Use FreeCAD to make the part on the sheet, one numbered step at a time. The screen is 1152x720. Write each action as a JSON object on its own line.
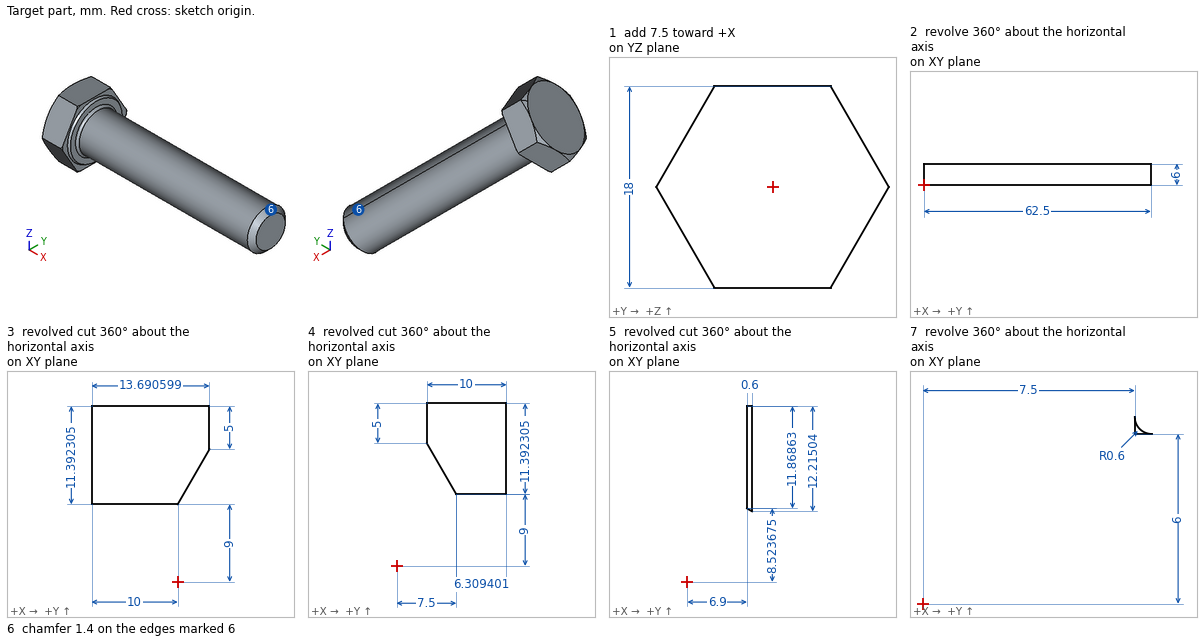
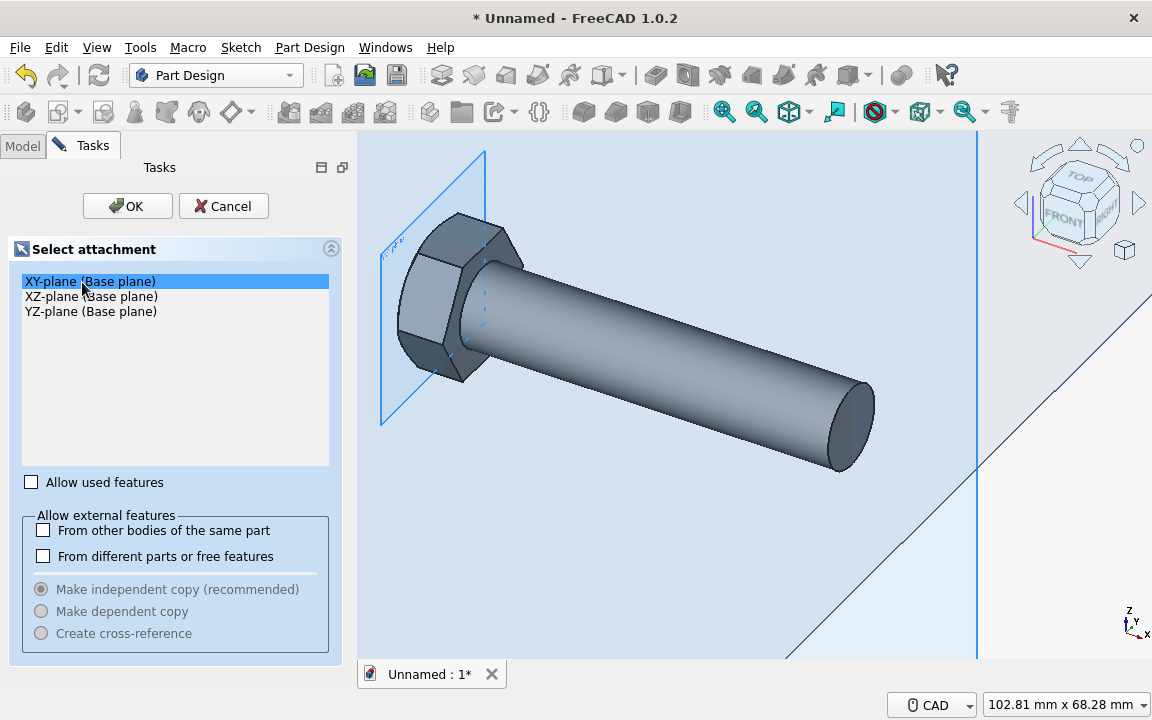
{"action": "left_click", "coordinate": [128, 206]}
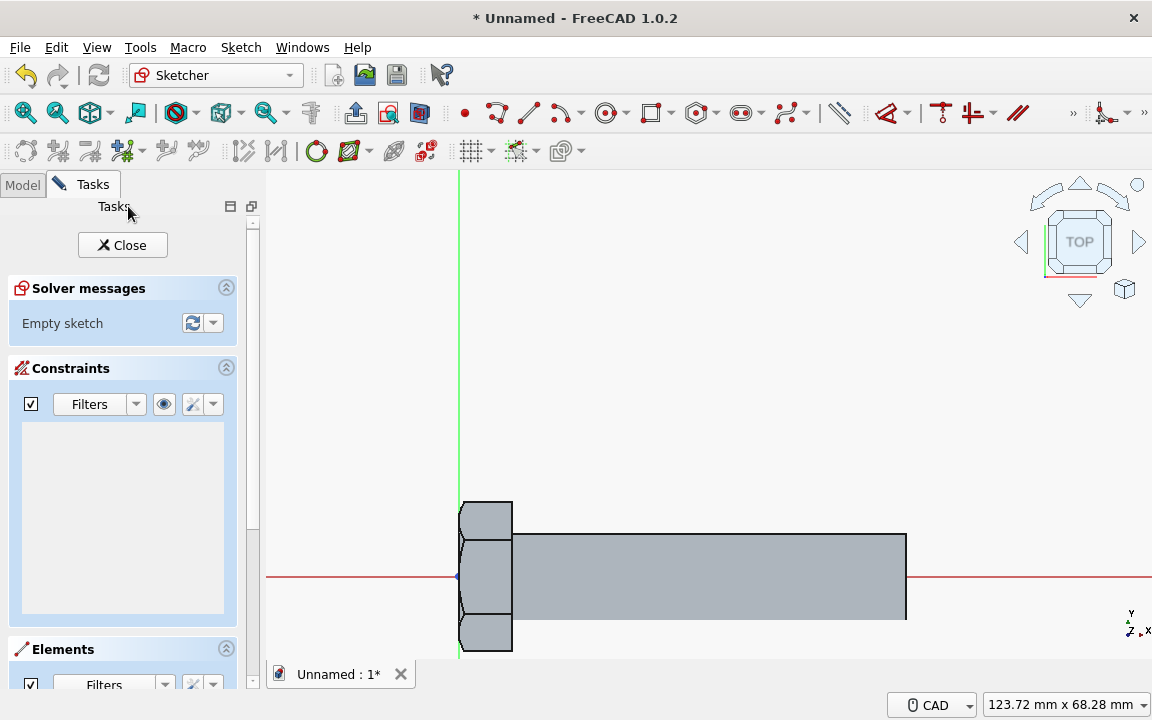
{"action": "key", "text": "q s"}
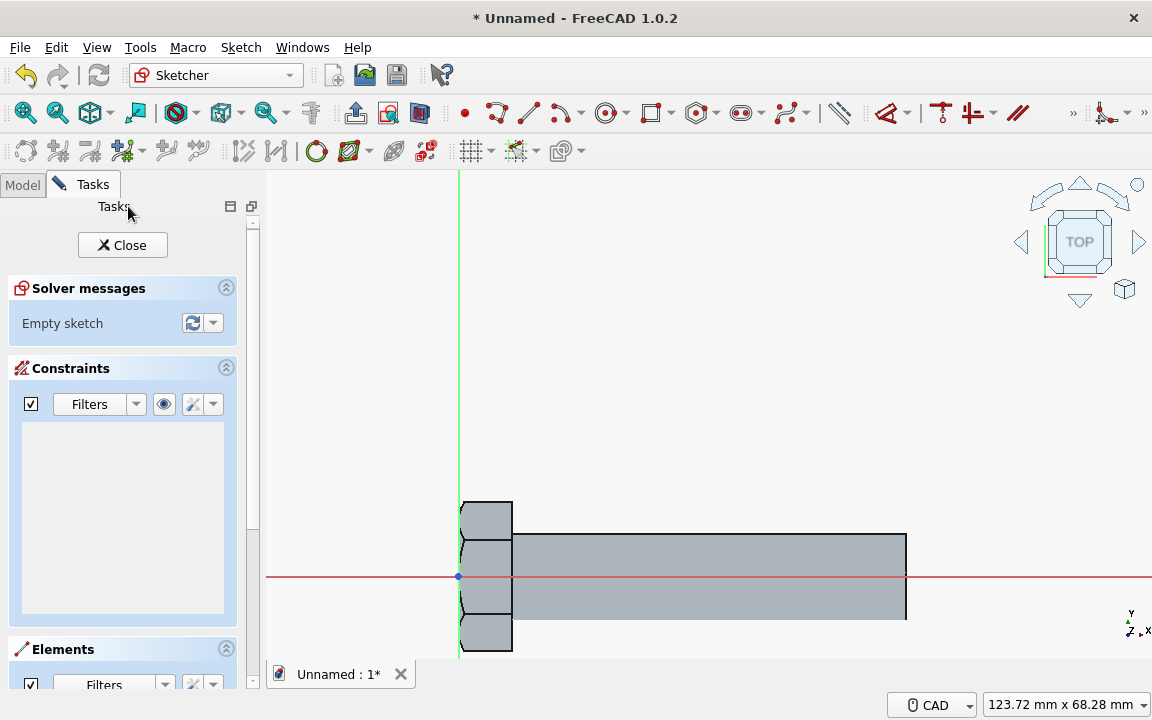
{"action": "scroll", "coordinate": [400, 577], "scroll_direction": "up", "scroll_amount": 4}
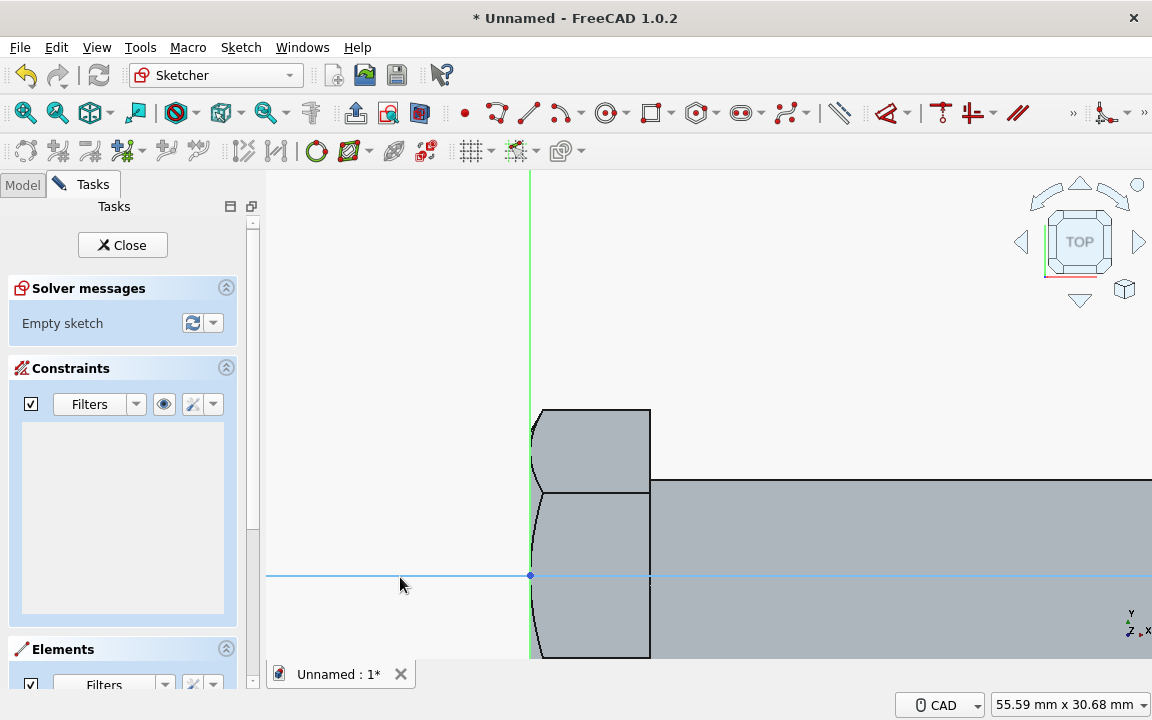
{"action": "key", "text": "g m"}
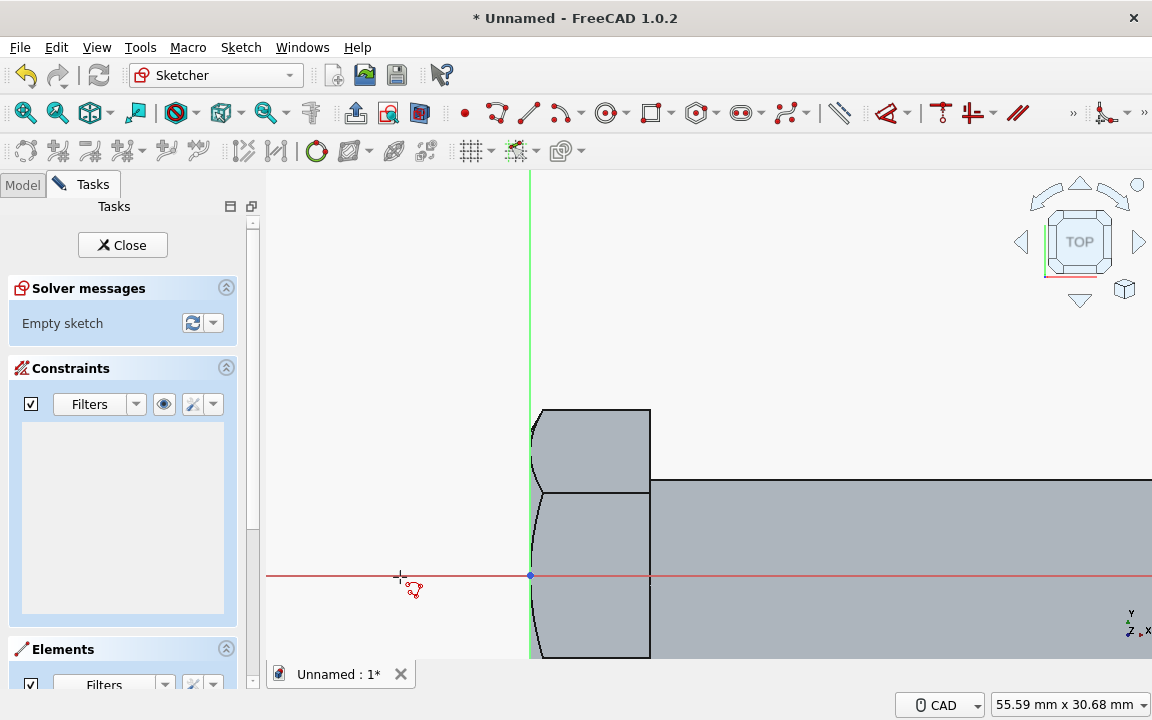
{"action": "left_click", "coordinate": [650, 432]}
{"action": "left_click", "coordinate": [750, 432]}
{"action": "left_click", "coordinate": [750, 251]}
{"action": "left_click", "coordinate": [591, 251]}
{"action": "left_click", "coordinate": [591, 330]}
{"action": "left_click", "coordinate": [650, 433]}
{"action": "key", "text": "Escape"}
{"action": "key", "text": "Escape"}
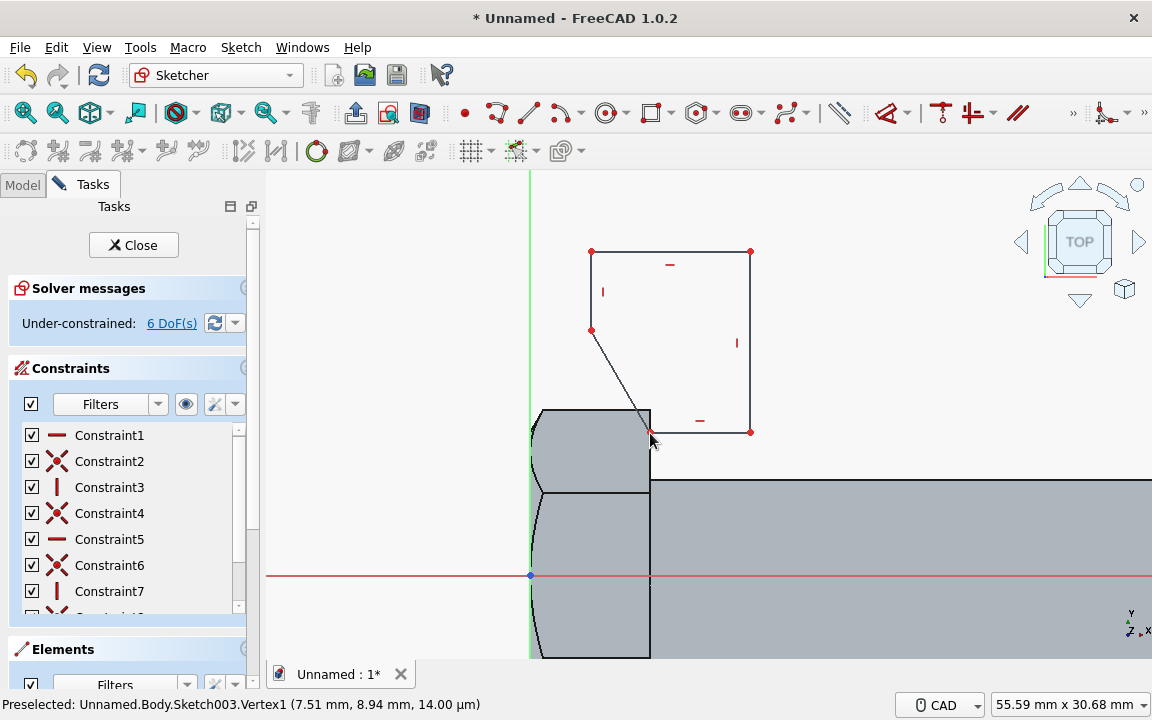
{"action": "key", "text": "d"}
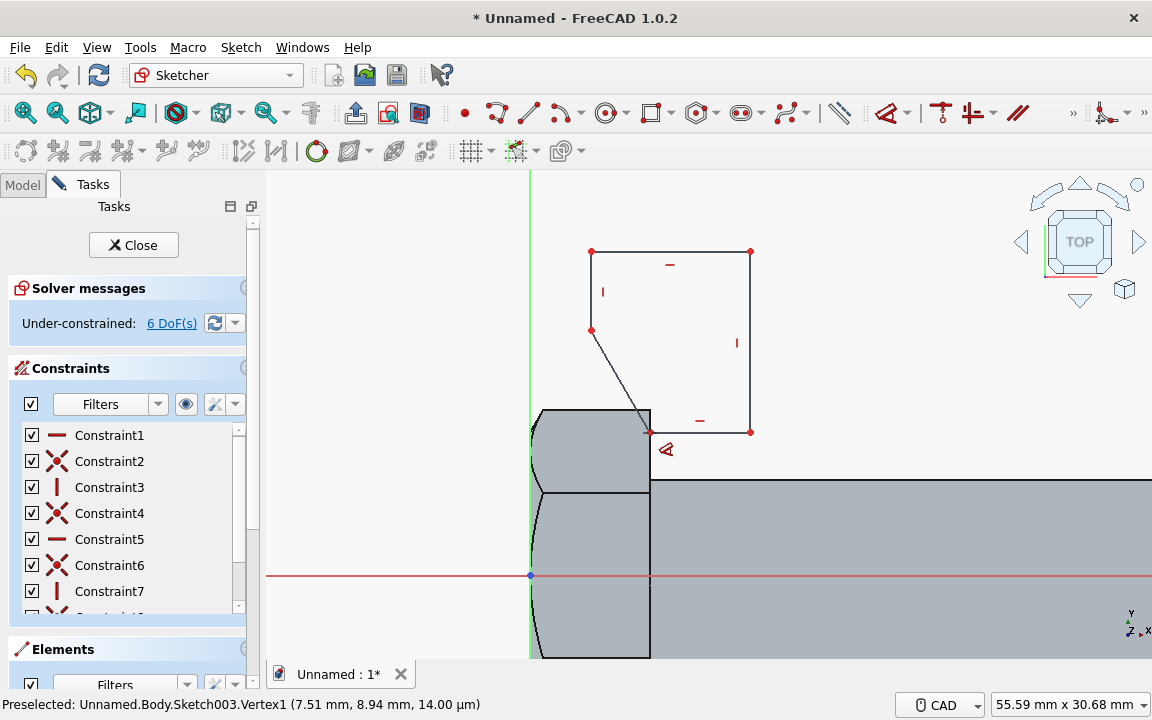
{"action": "left_click", "coordinate": [591, 276]}
{"action": "left_click", "coordinate": [557, 291]}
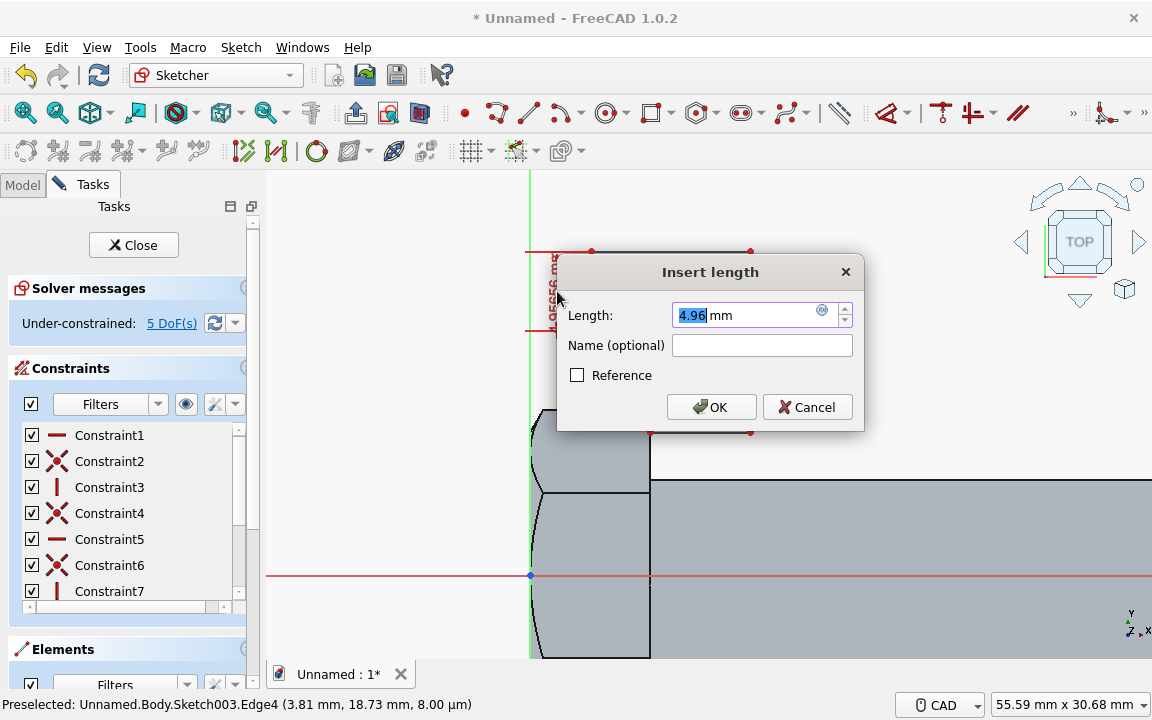
{"action": "type", "text": "5"}
{"action": "key", "text": "Return"}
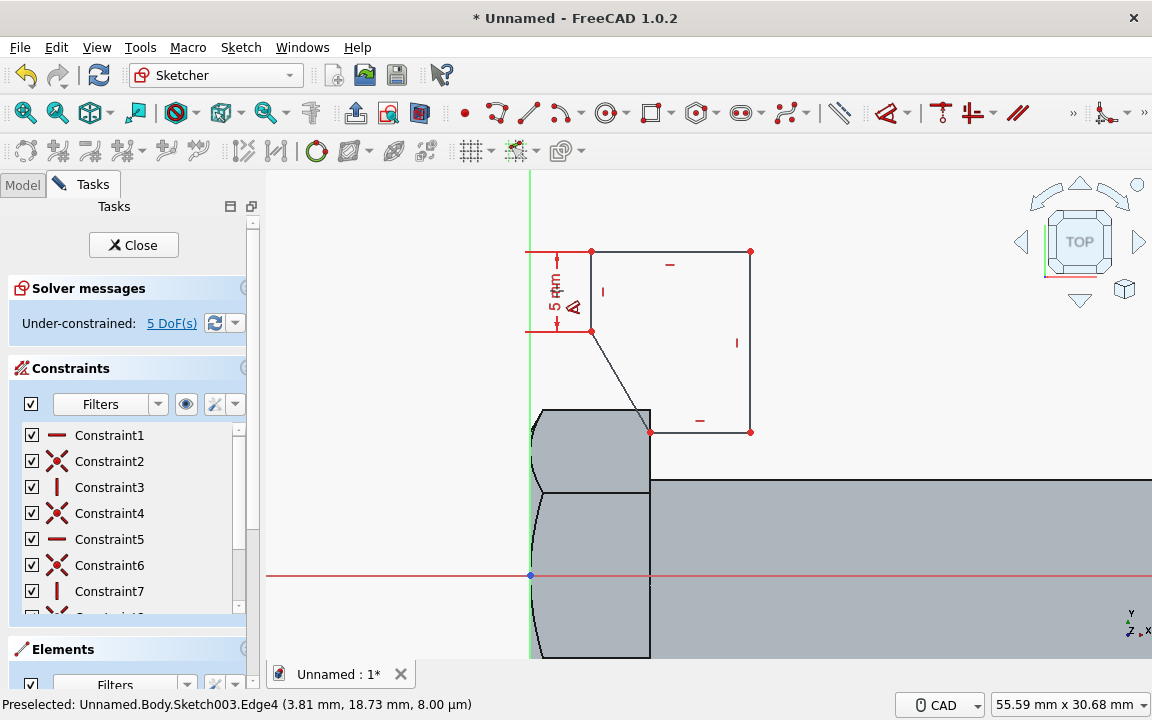
{"action": "left_click", "coordinate": [702, 252]}
{"action": "left_click", "coordinate": [670, 218]}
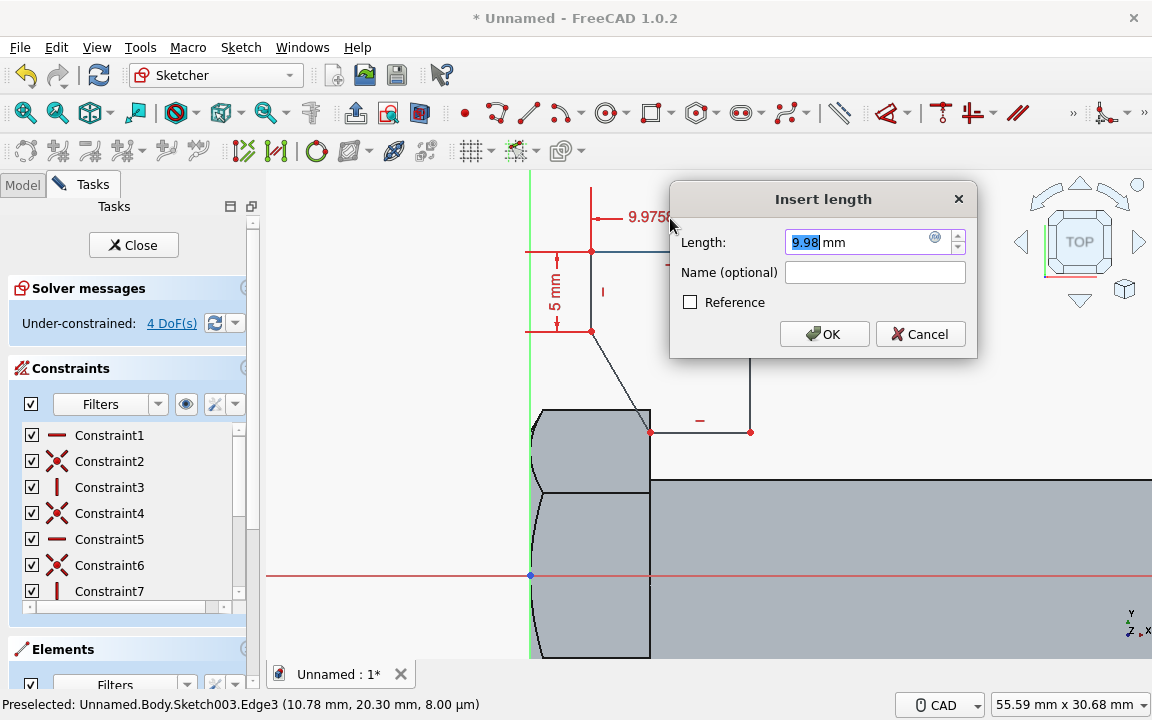
{"action": "type", "text": "10"}
{"action": "key", "text": "Return"}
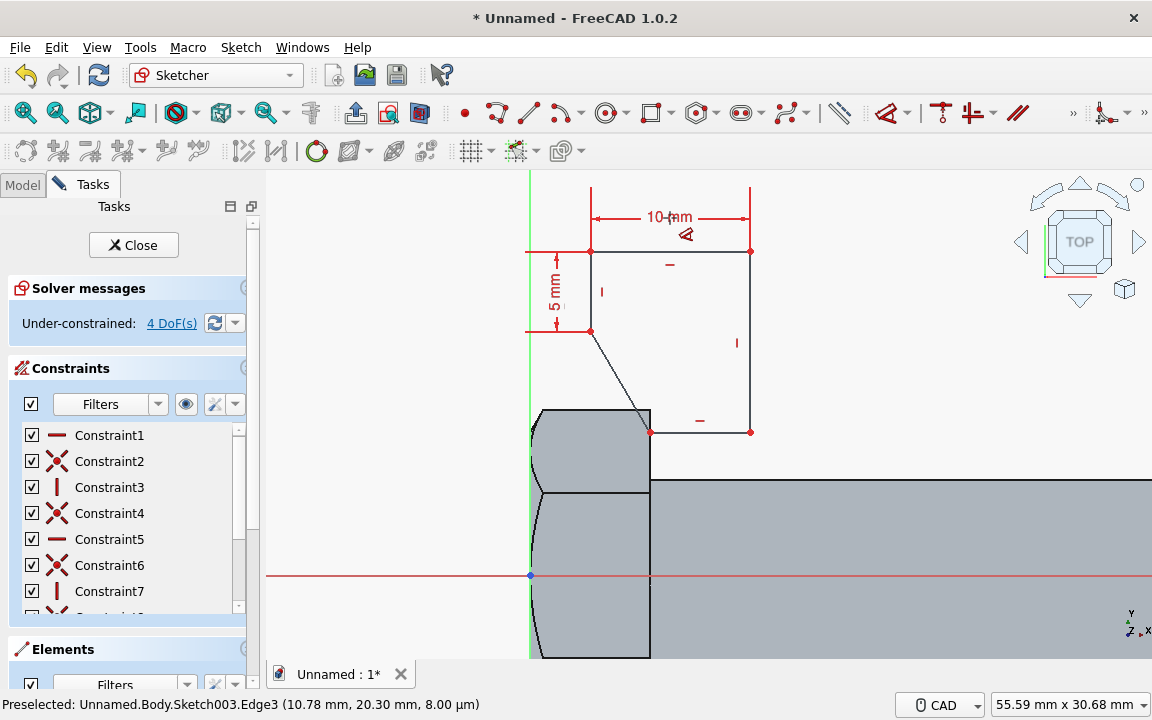
{"action": "left_click", "coordinate": [650, 433]}
{"action": "left_click", "coordinate": [496, 504]}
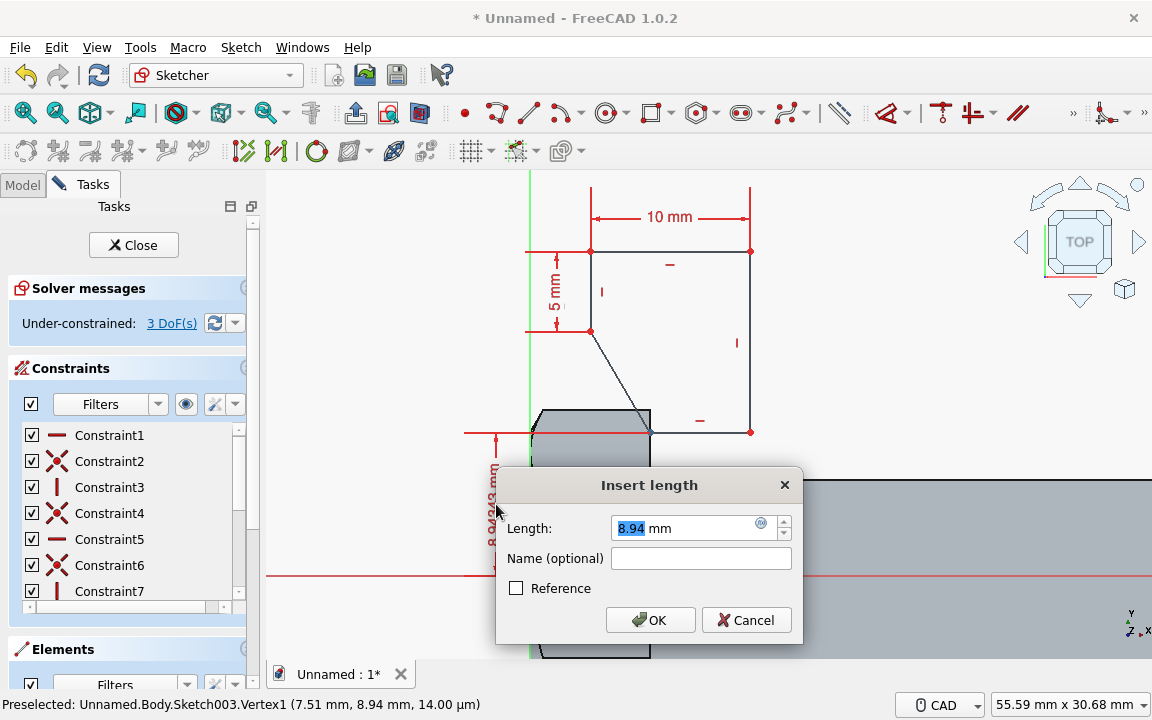
{"action": "type", "text": "9"}
{"action": "key", "text": "Return"}